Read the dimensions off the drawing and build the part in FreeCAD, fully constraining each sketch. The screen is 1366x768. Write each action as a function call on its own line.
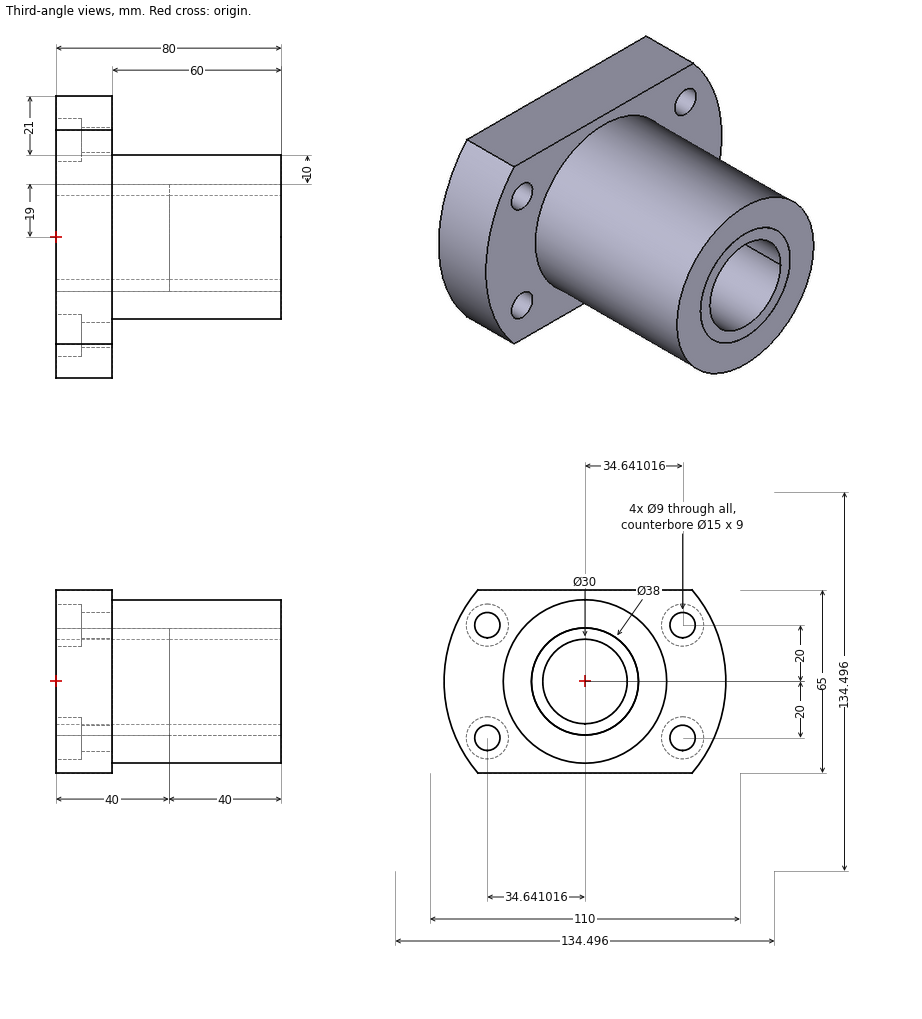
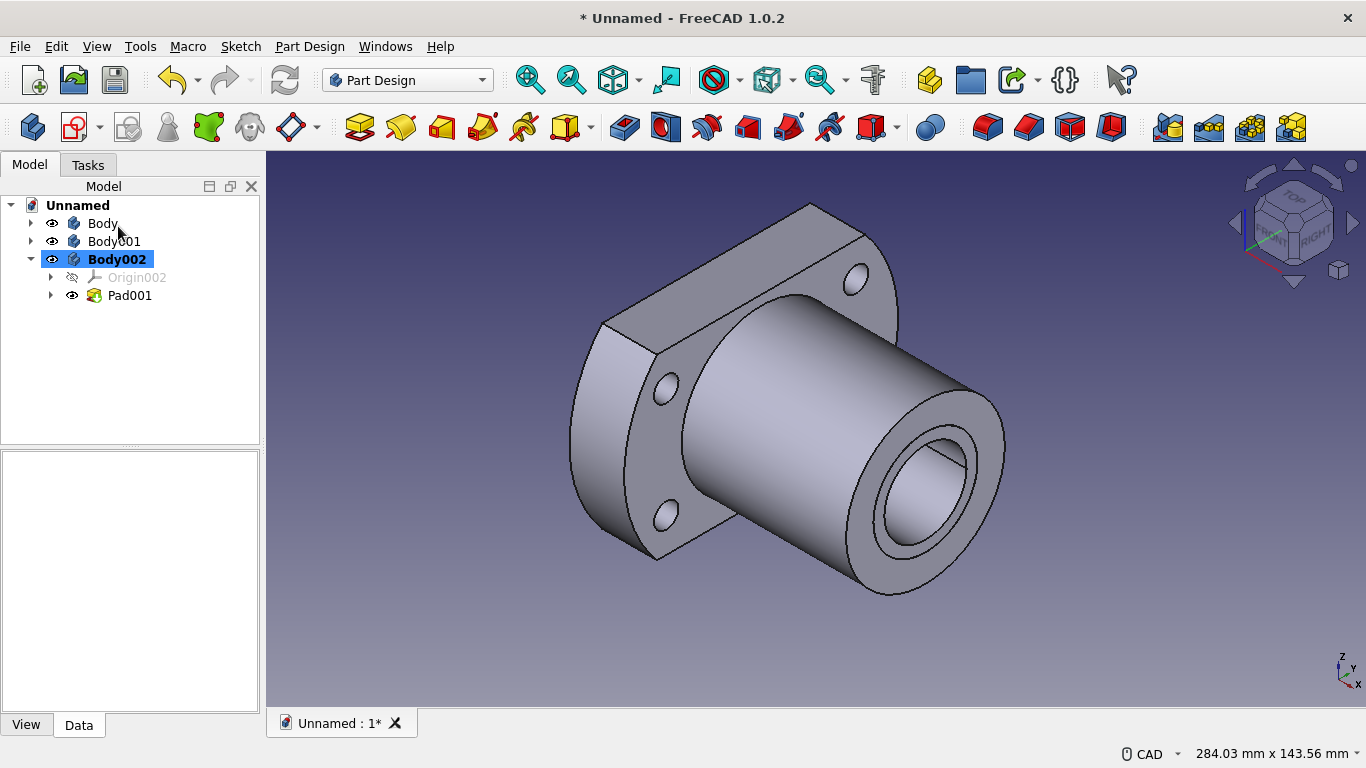
click(531, 80)